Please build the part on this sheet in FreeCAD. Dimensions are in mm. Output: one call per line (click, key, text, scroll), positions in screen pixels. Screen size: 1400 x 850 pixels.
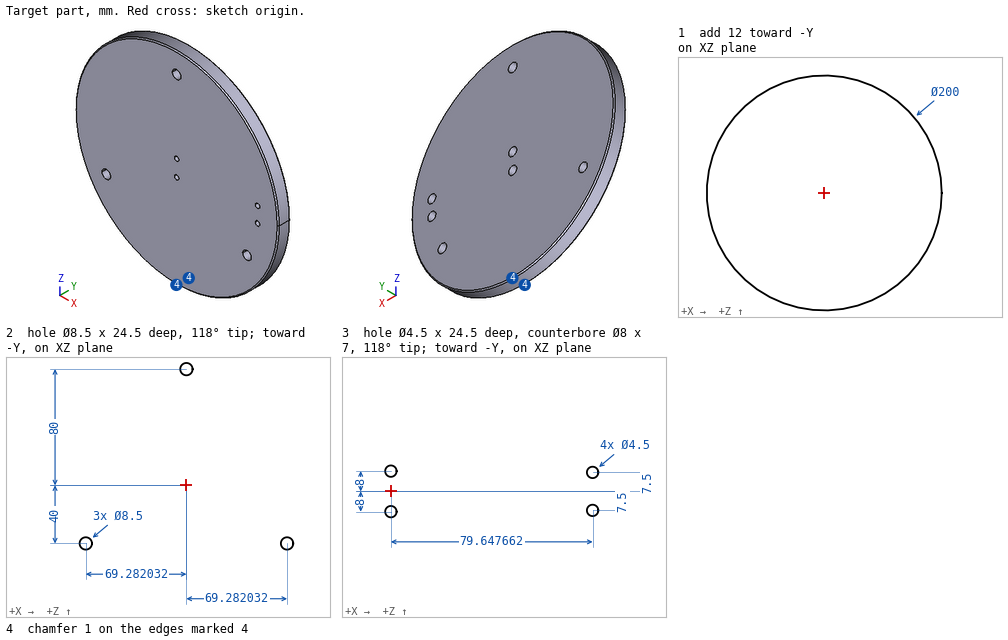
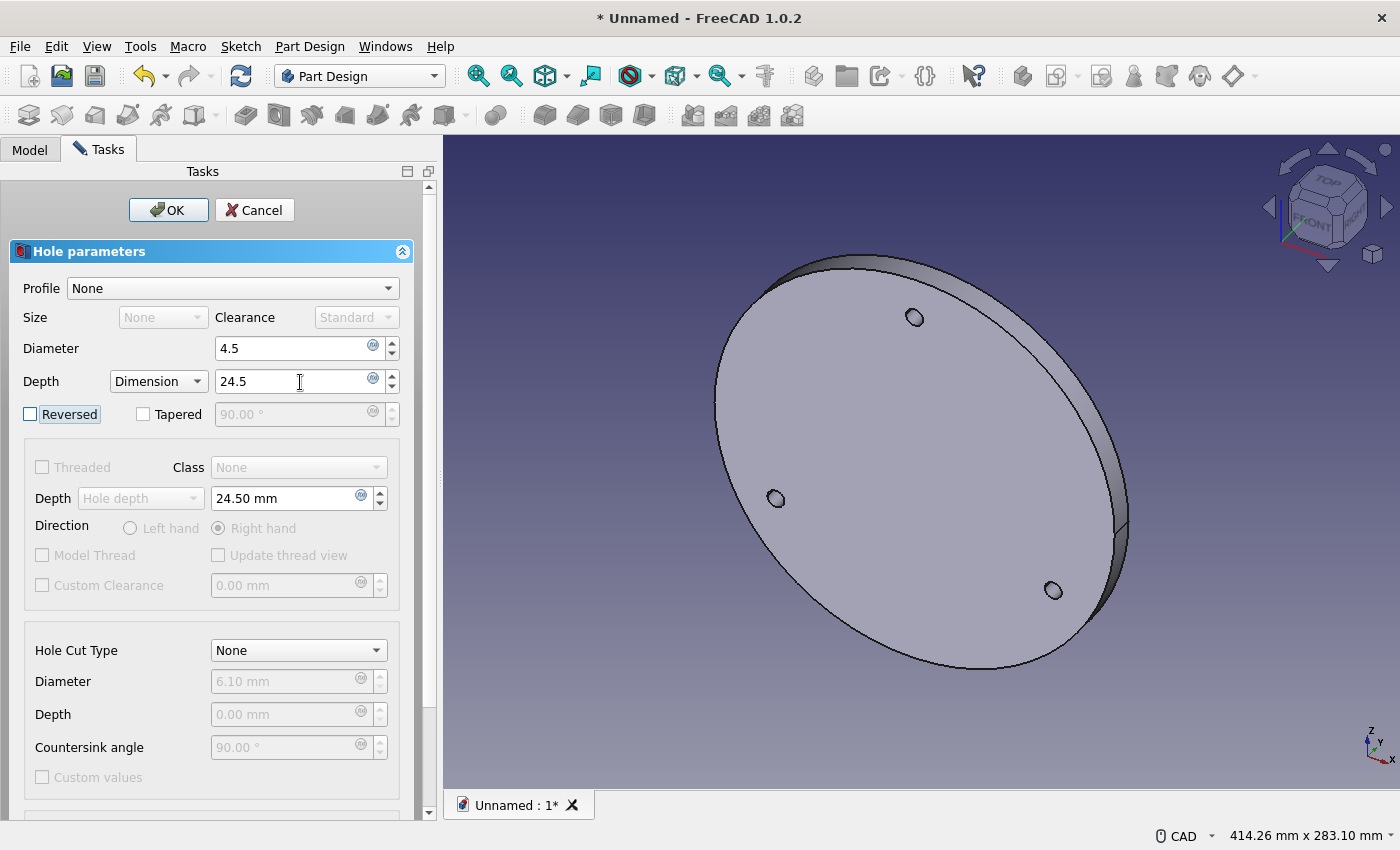
click(31, 414)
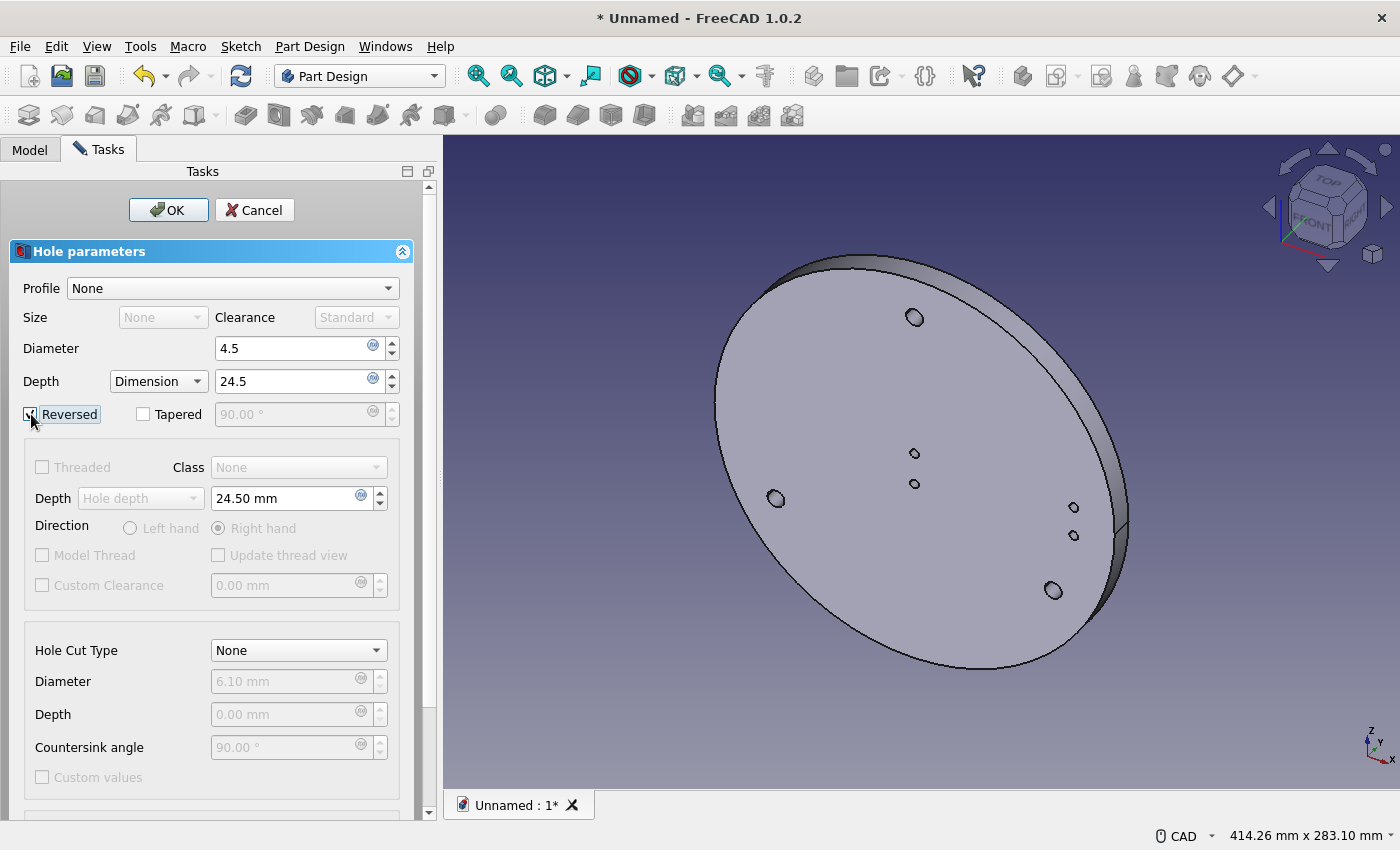
click(300, 650)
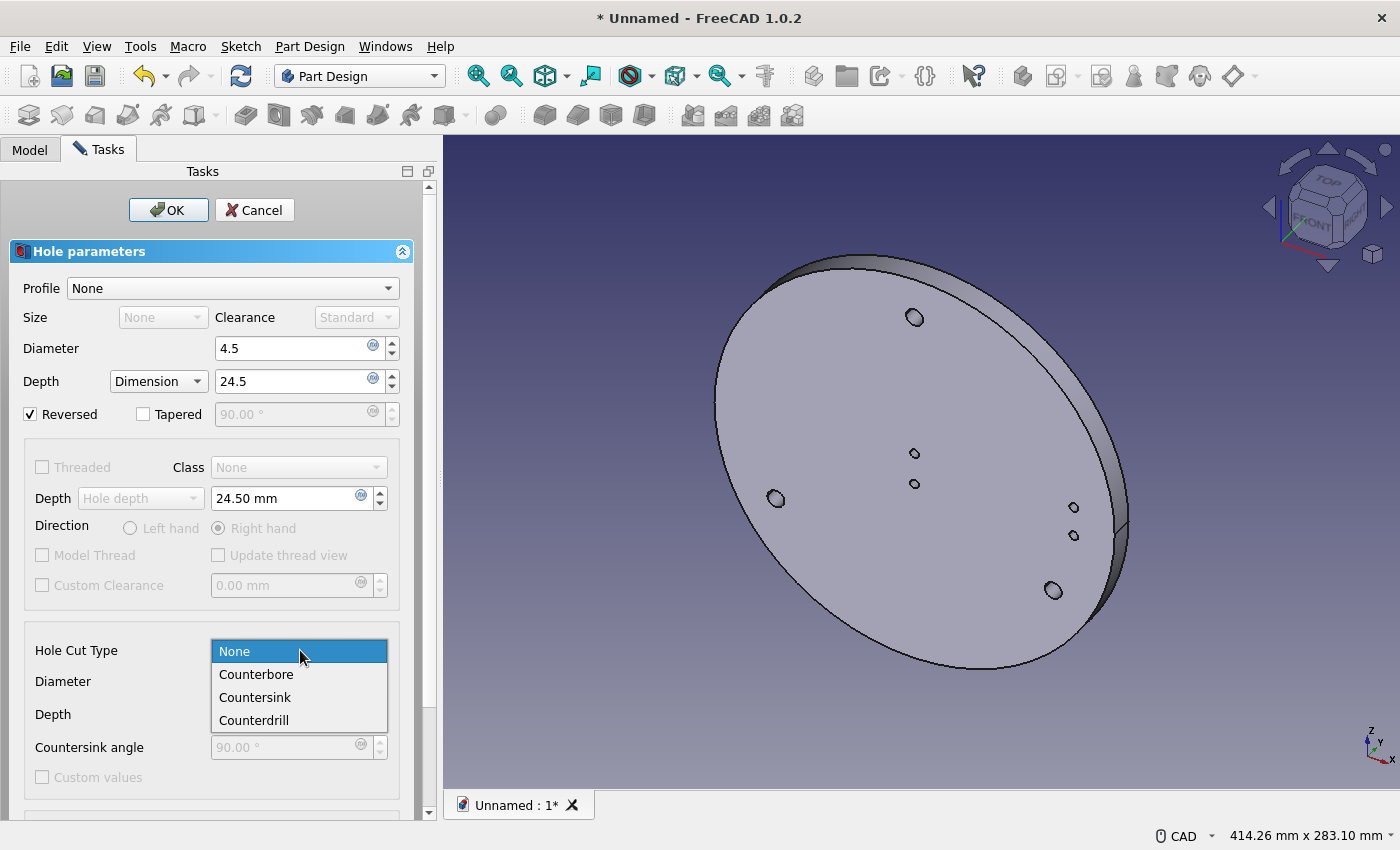
click(298, 674)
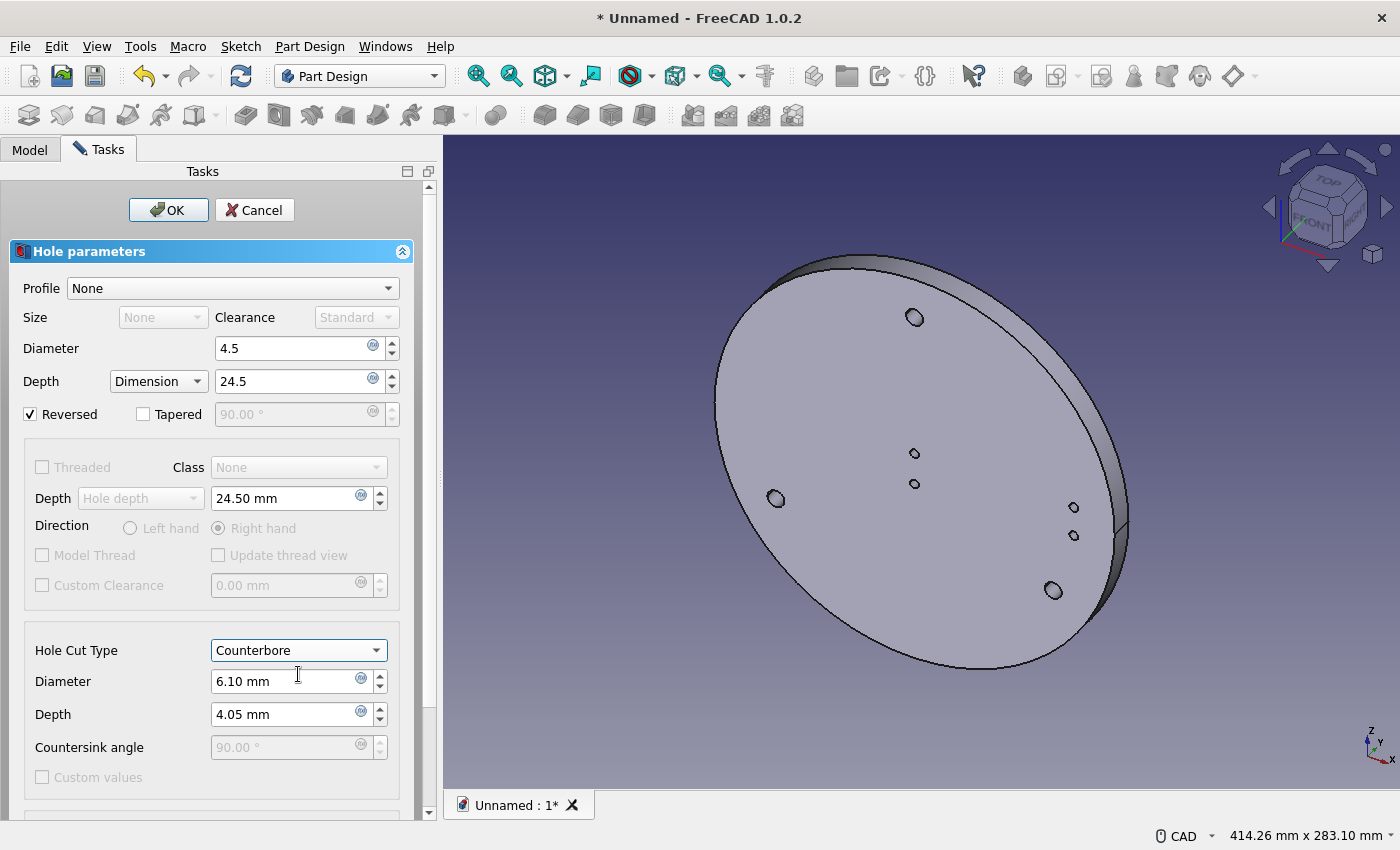
triple_click(292, 682)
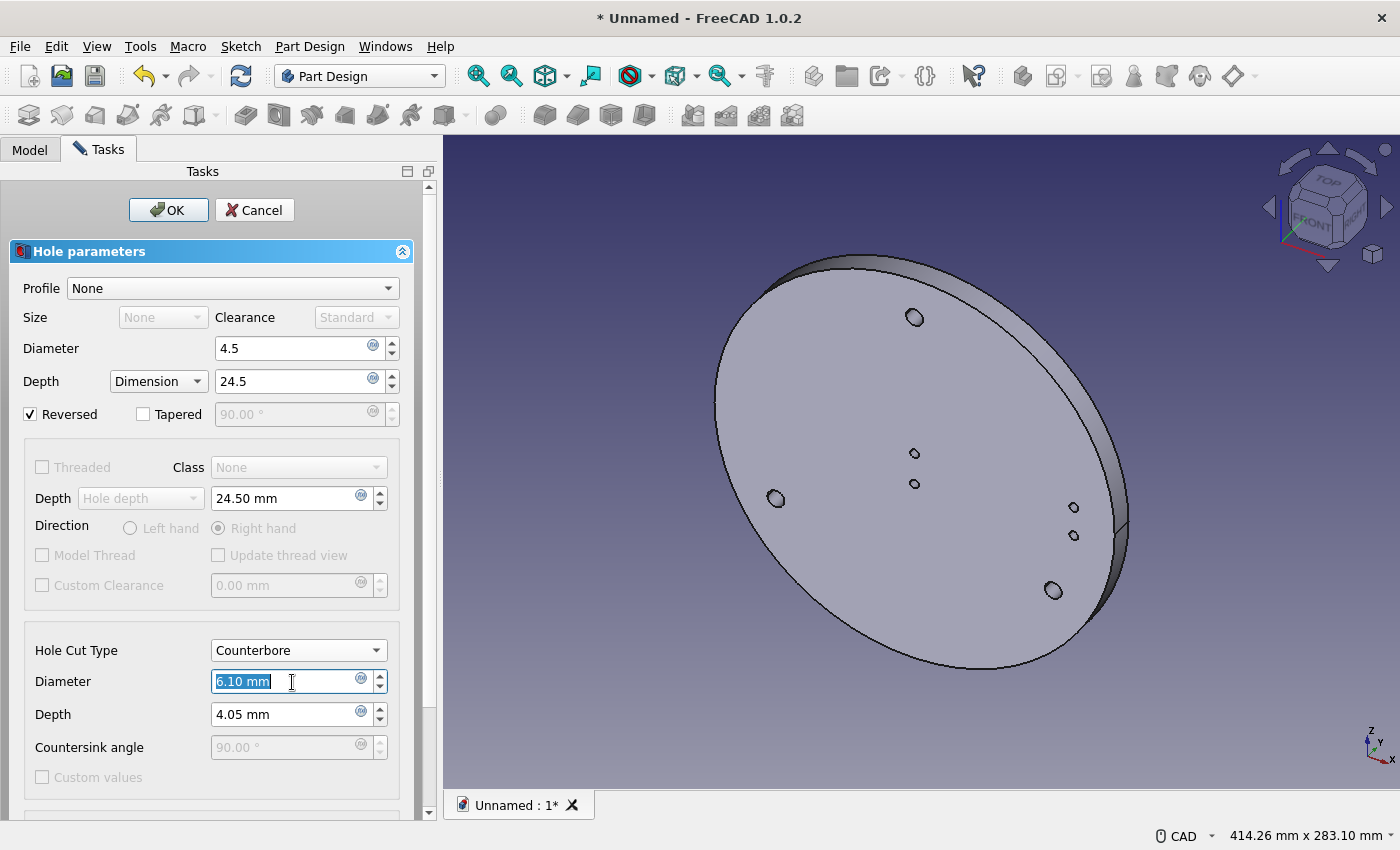
text(8)
key(Tab)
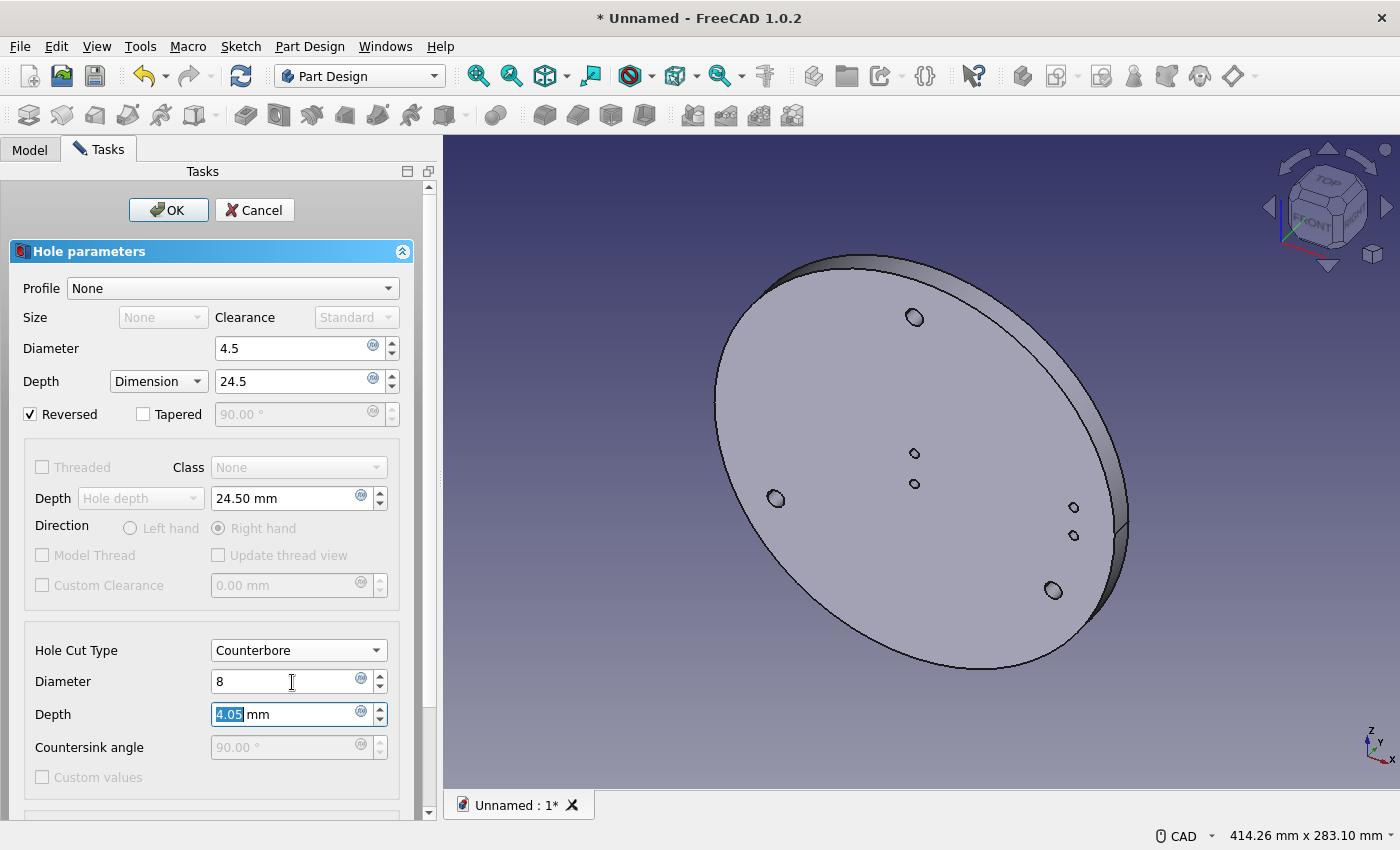
text(7)
key(Tab)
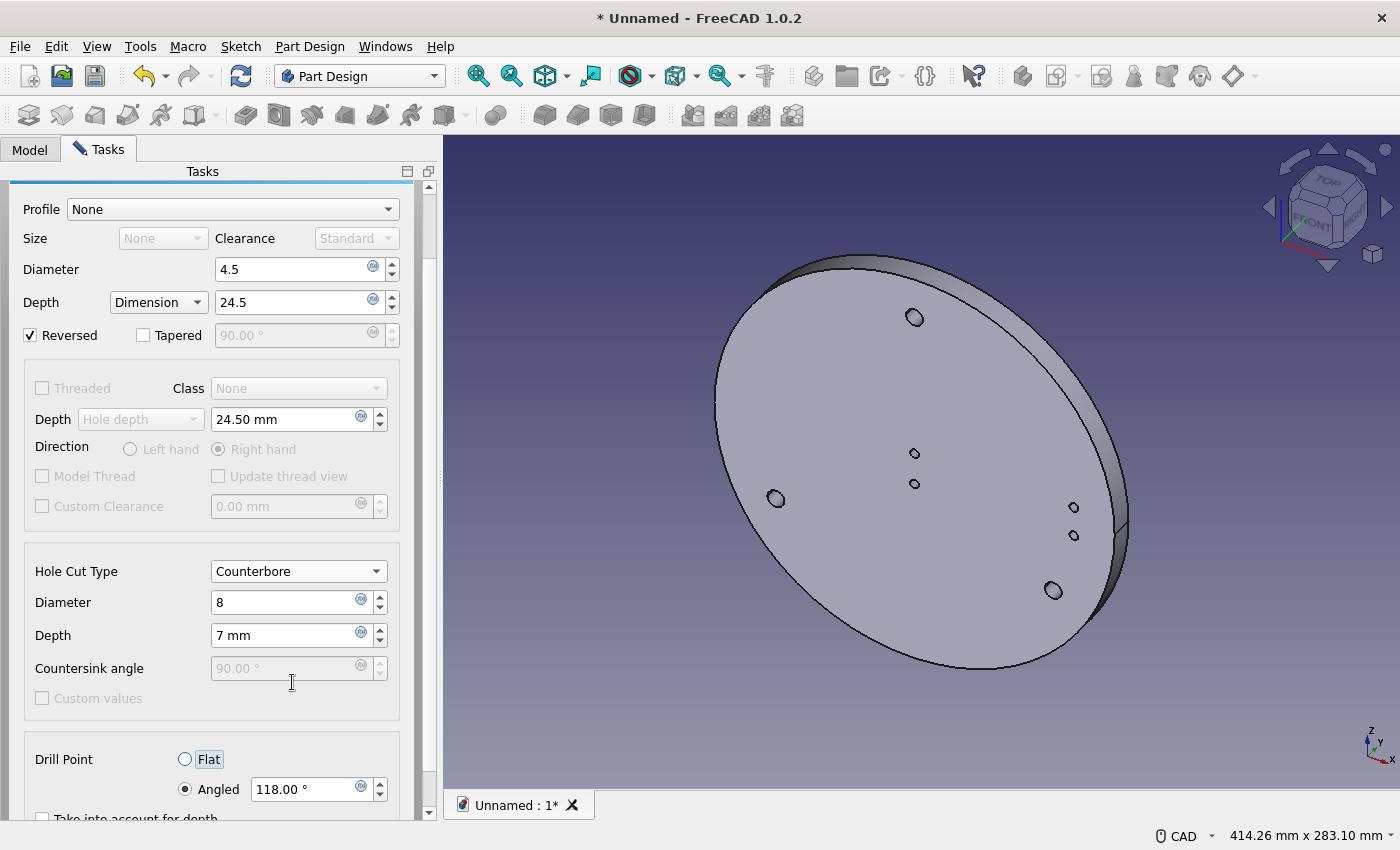
scroll(429, 500, up, 3)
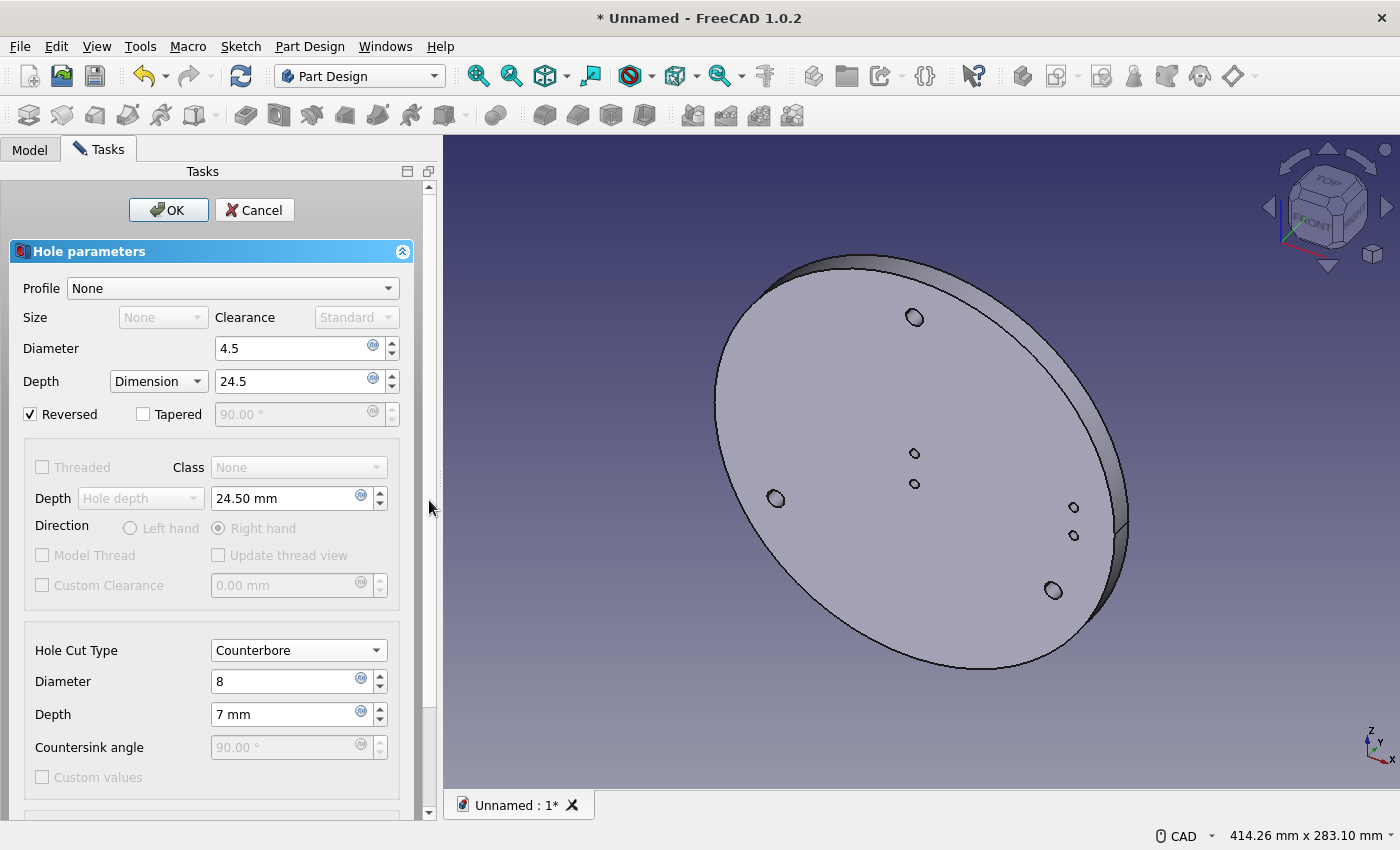
click(169, 210)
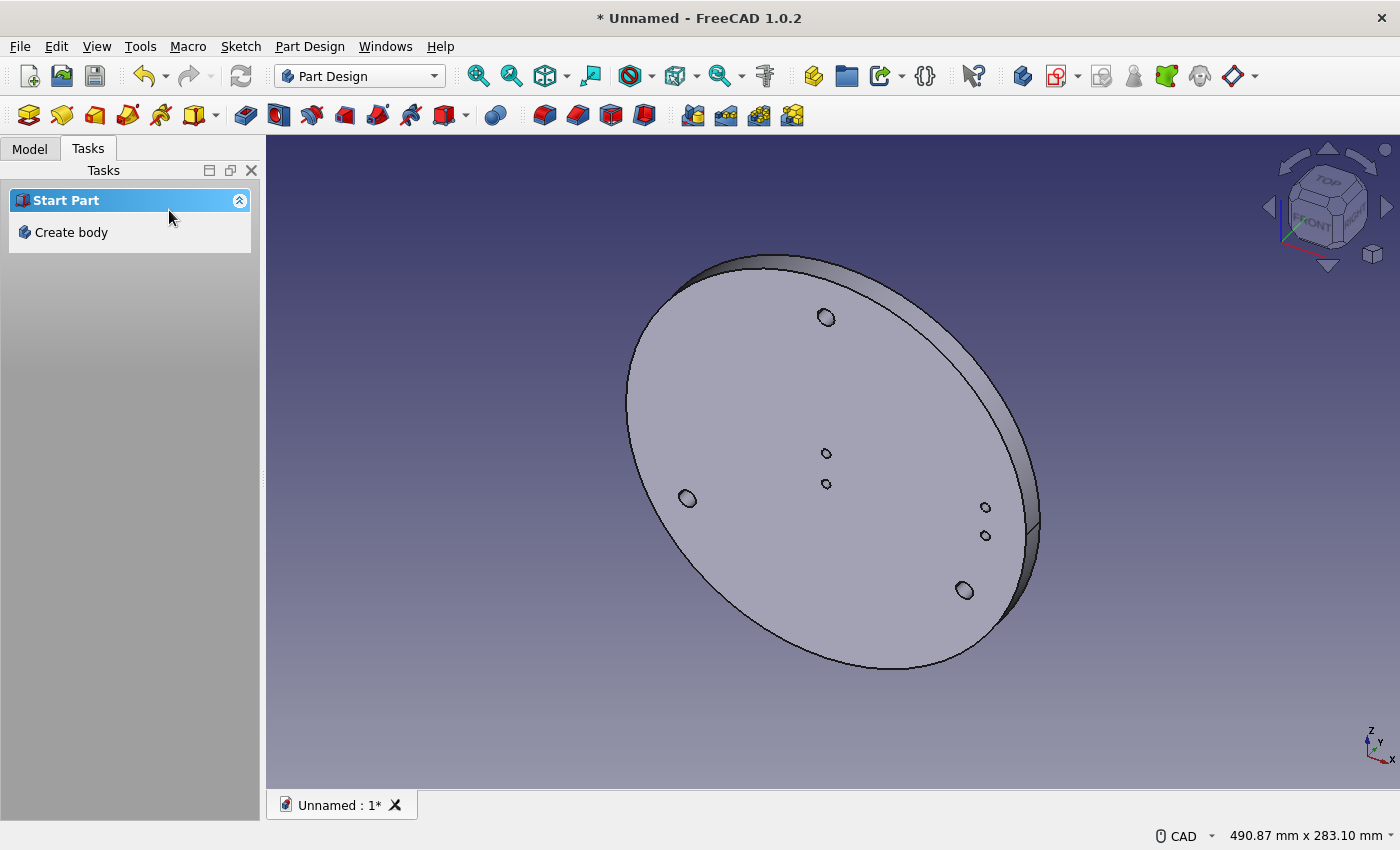
click(664, 303)